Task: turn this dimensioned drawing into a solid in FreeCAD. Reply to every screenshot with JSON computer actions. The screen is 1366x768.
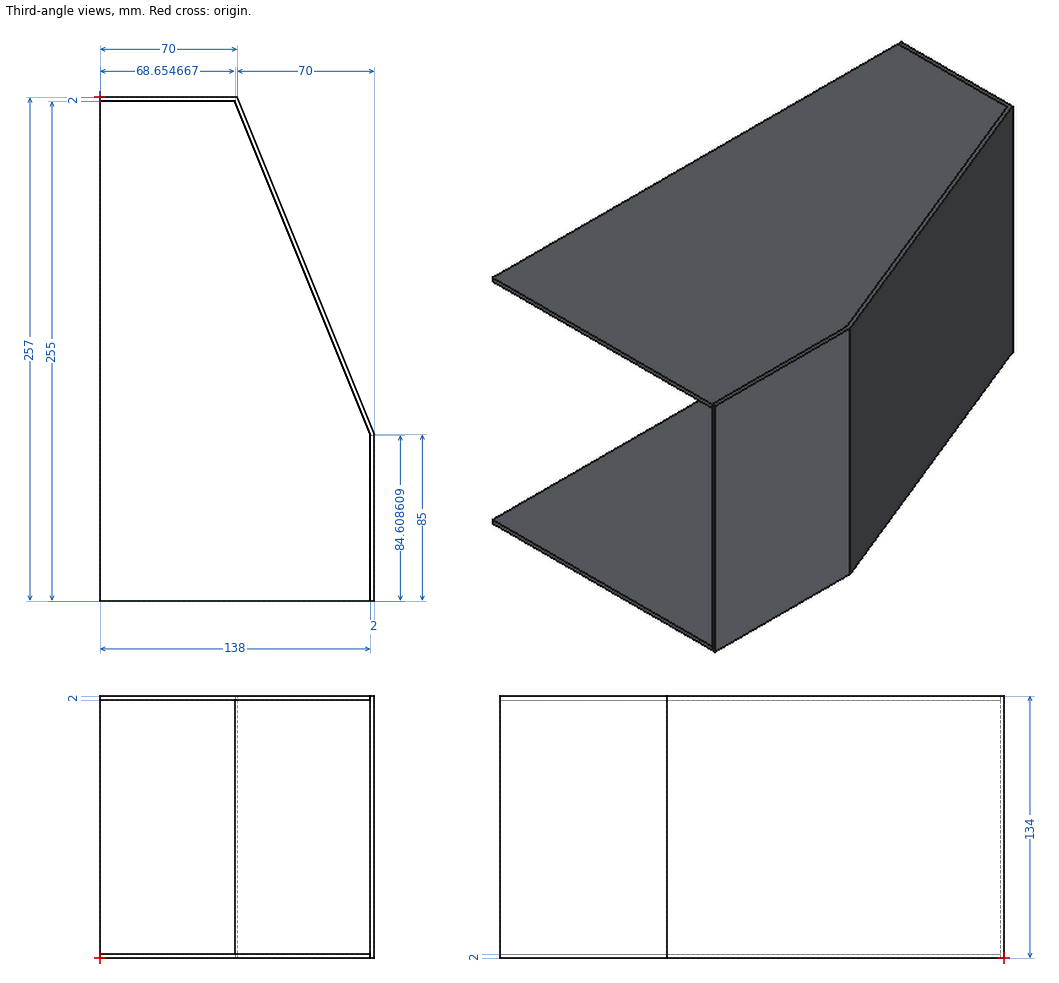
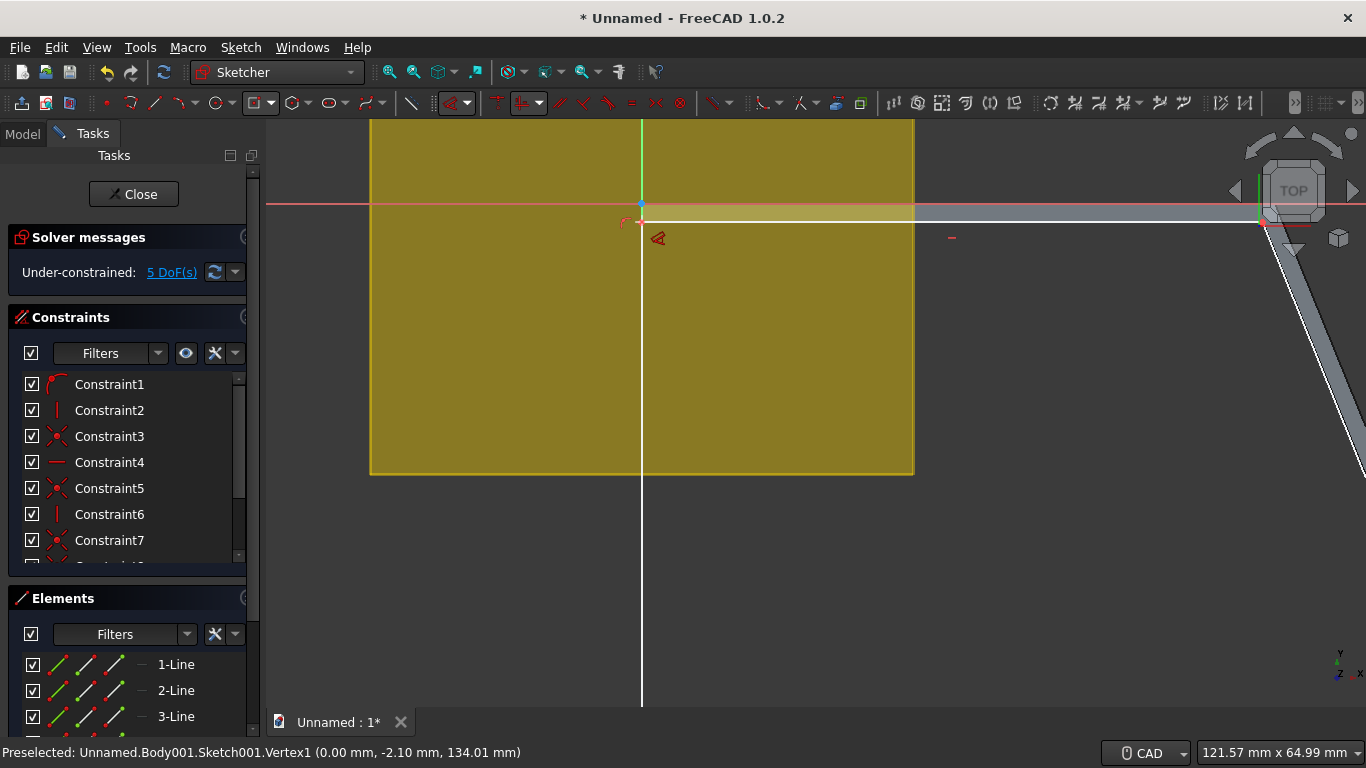
{"action": "scroll", "coordinate": [642, 222], "scroll_direction": "up", "scroll_amount": 4}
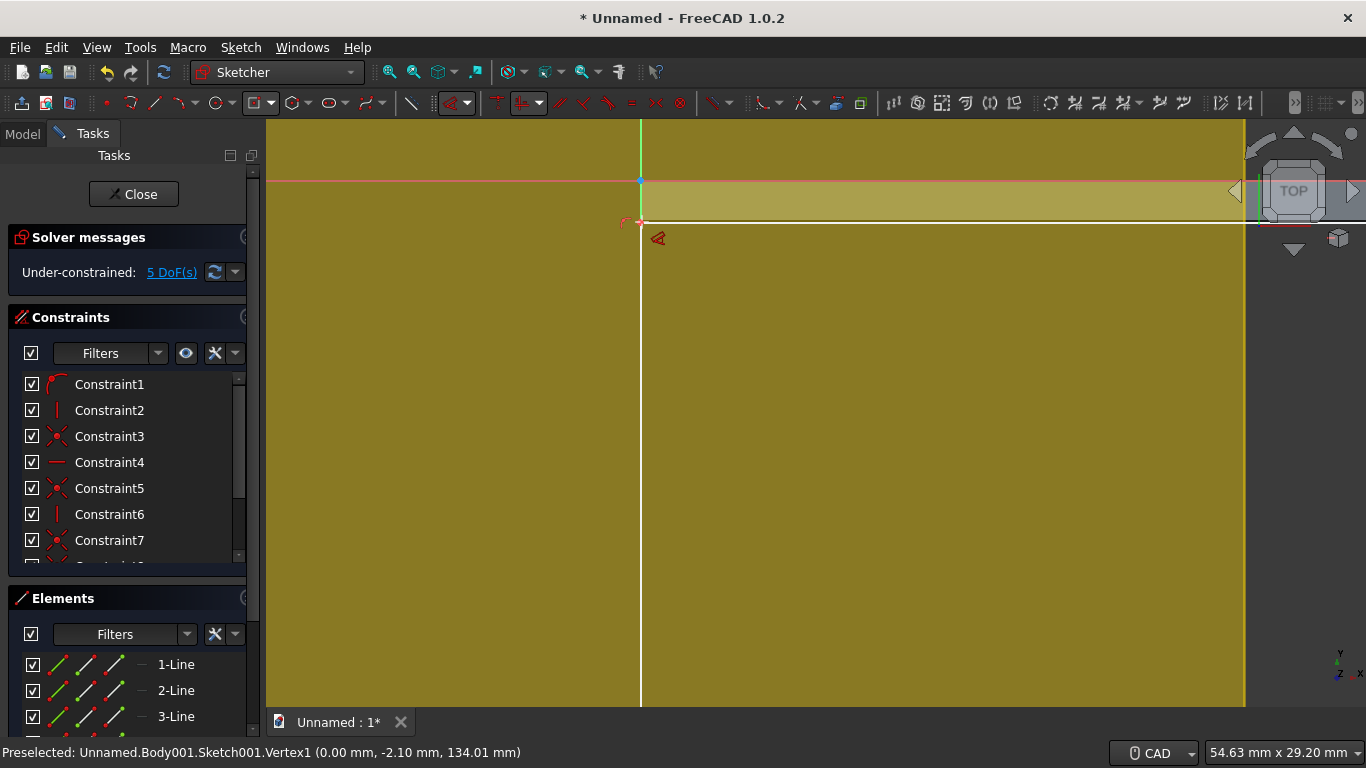
{"action": "left_click", "coordinate": [641, 223]}
{"action": "left_click", "coordinate": [607, 202]}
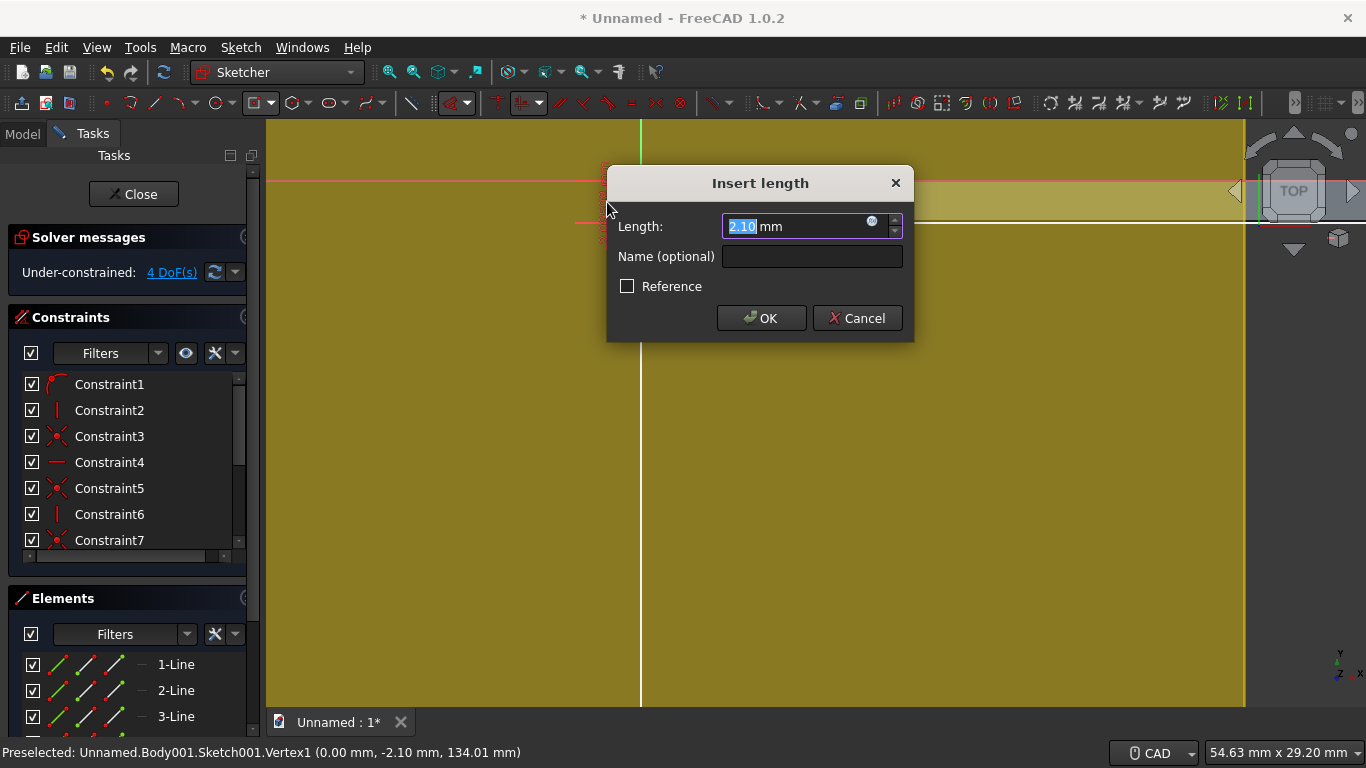
{"action": "type", "text": "2"}
{"action": "key", "text": "Return"}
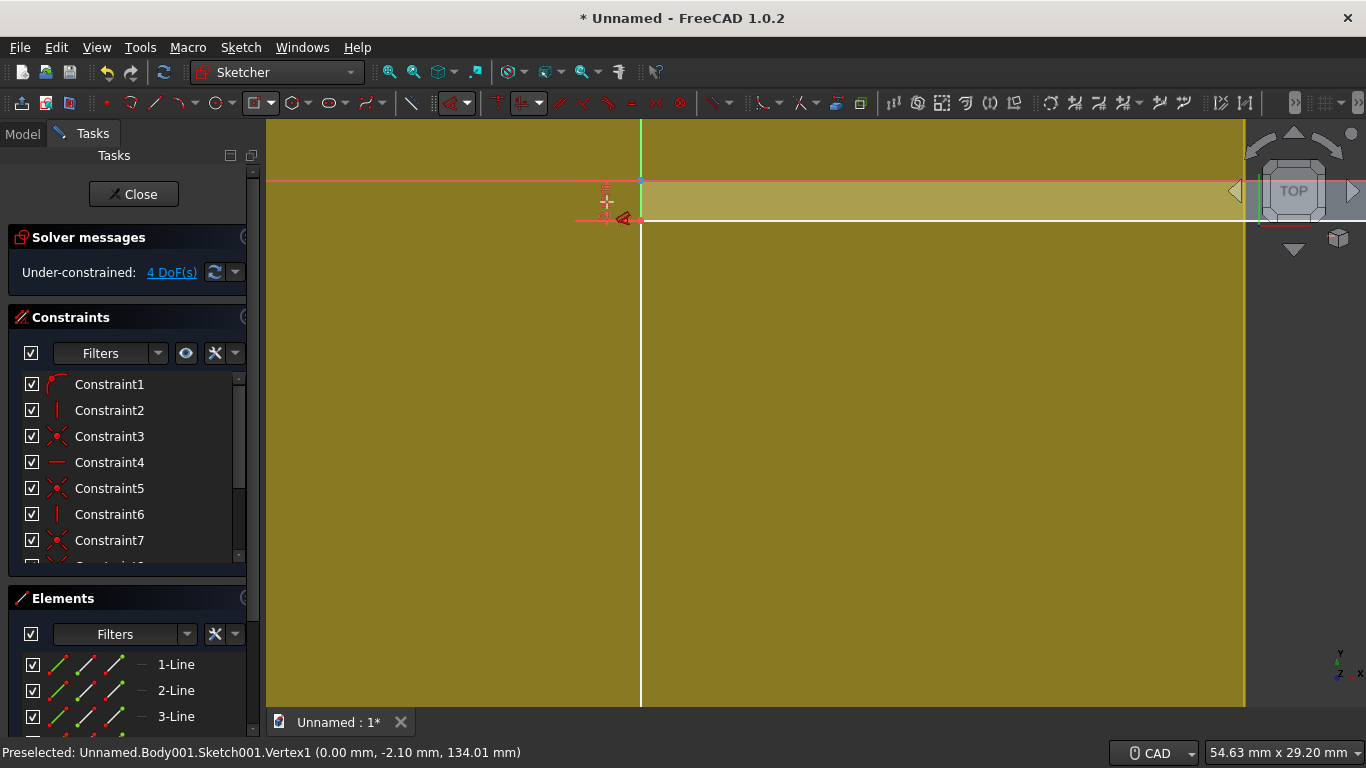
{"action": "scroll", "coordinate": [645, 224], "scroll_direction": "down", "scroll_amount": 13}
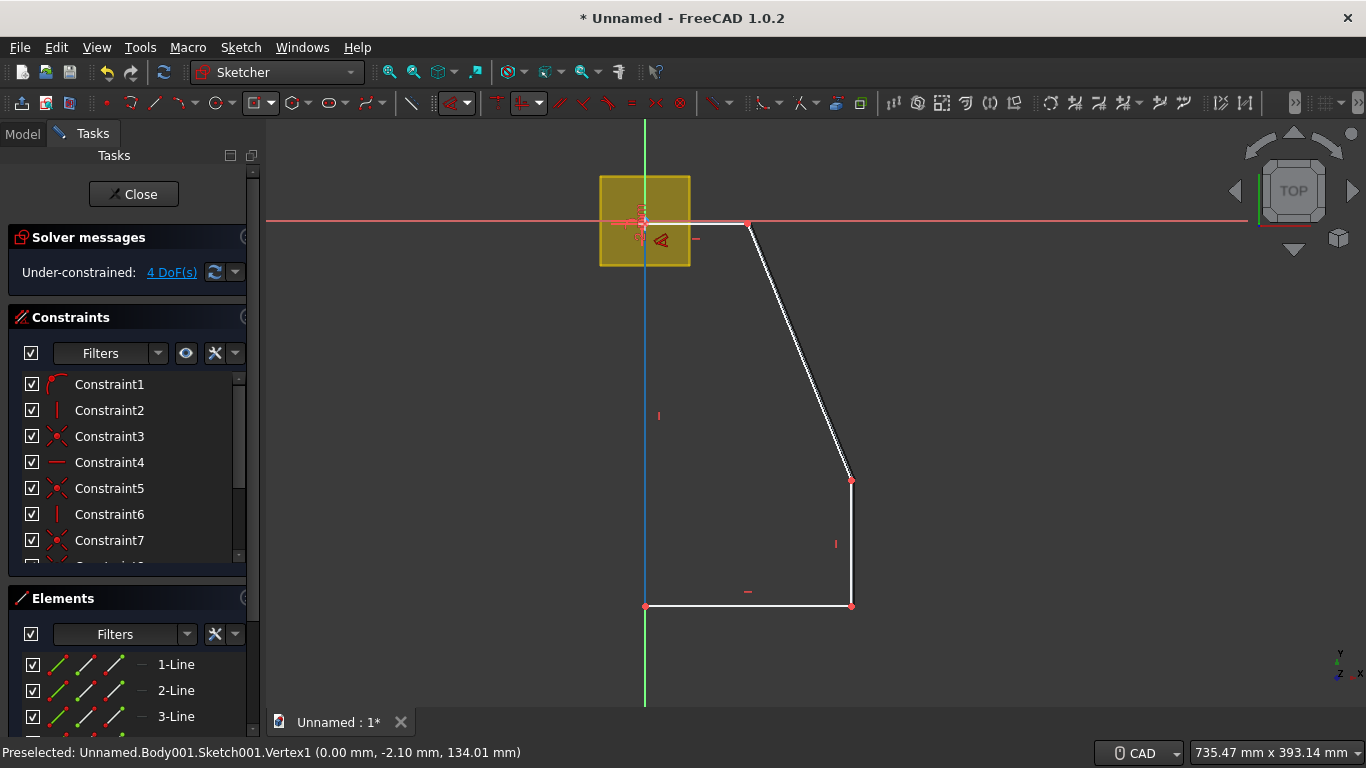
{"action": "left_click", "coordinate": [645, 339]}
{"action": "left_click", "coordinate": [611, 415]}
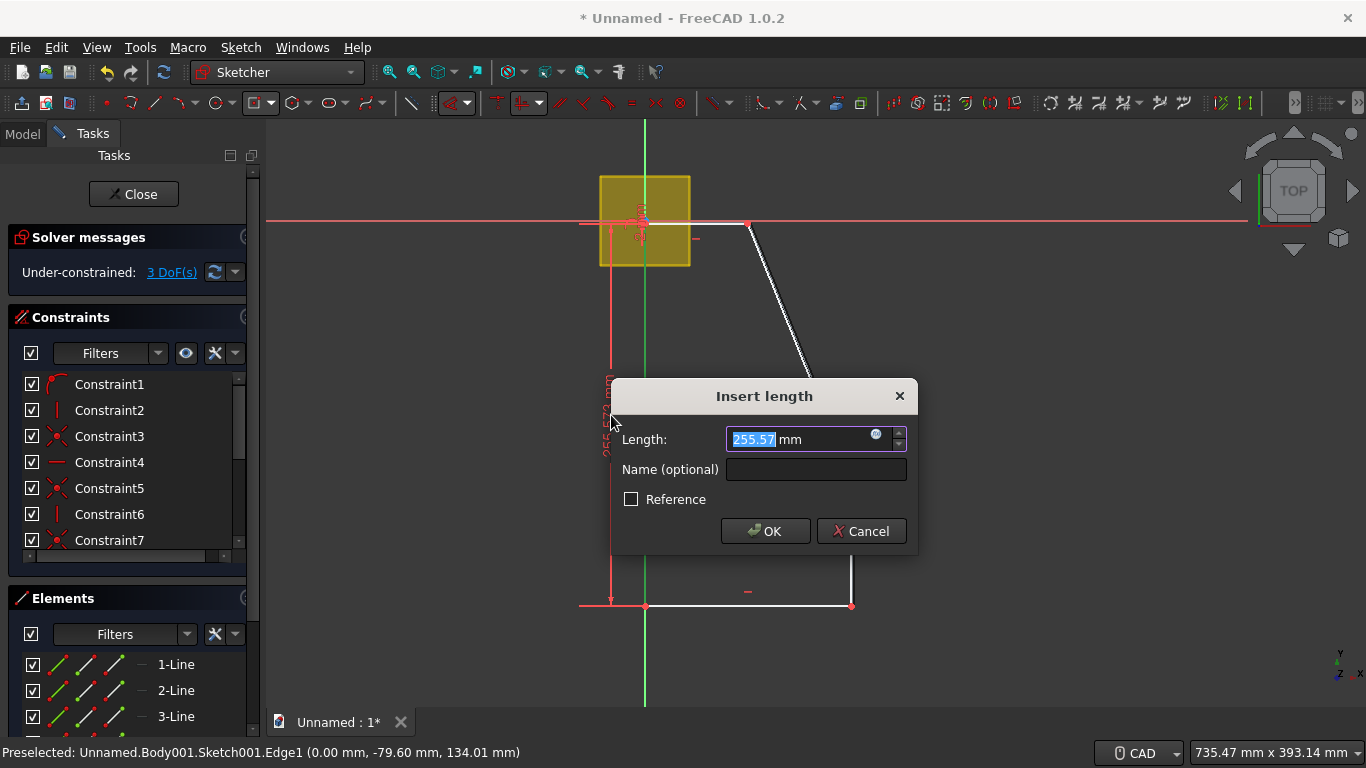
{"action": "type", "text": "255"}
{"action": "key", "text": "Return"}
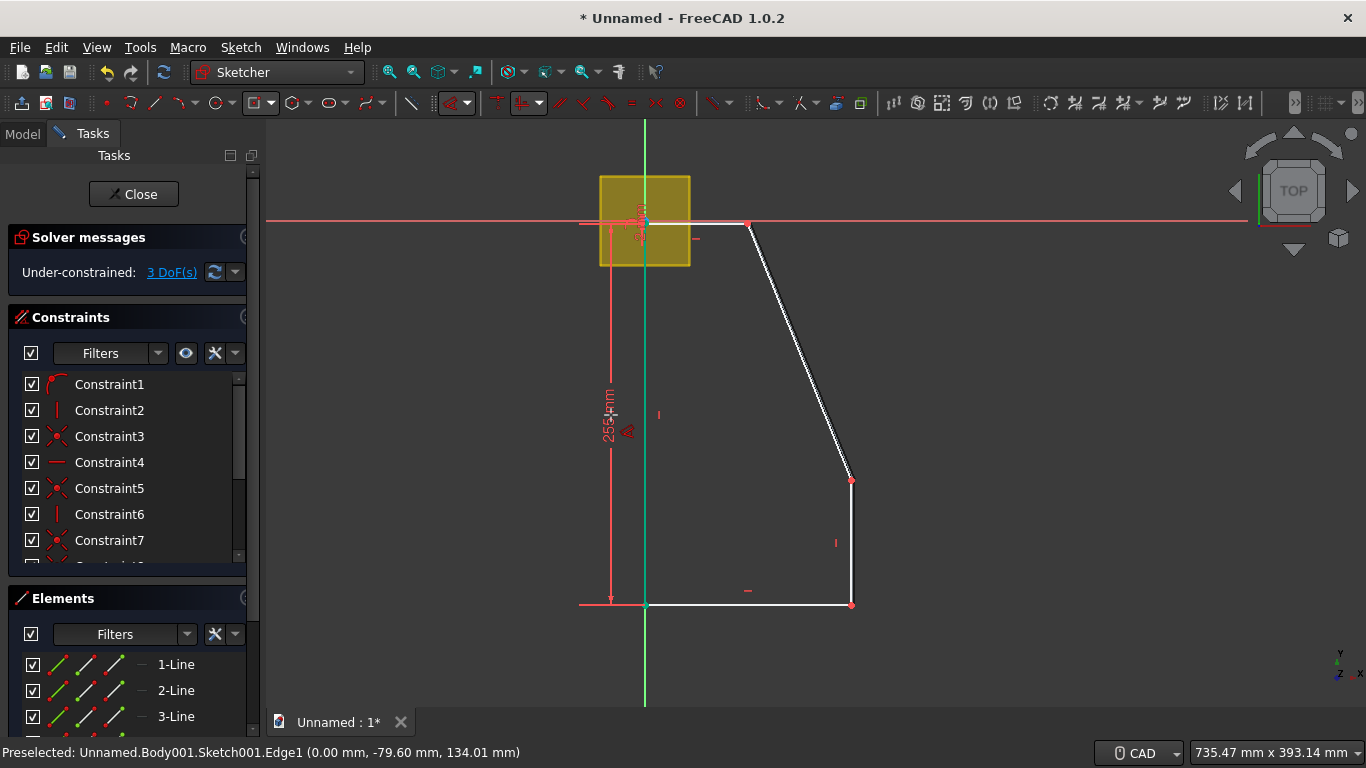
{"action": "left_click", "coordinate": [707, 605]}
{"action": "left_click", "coordinate": [748, 639]}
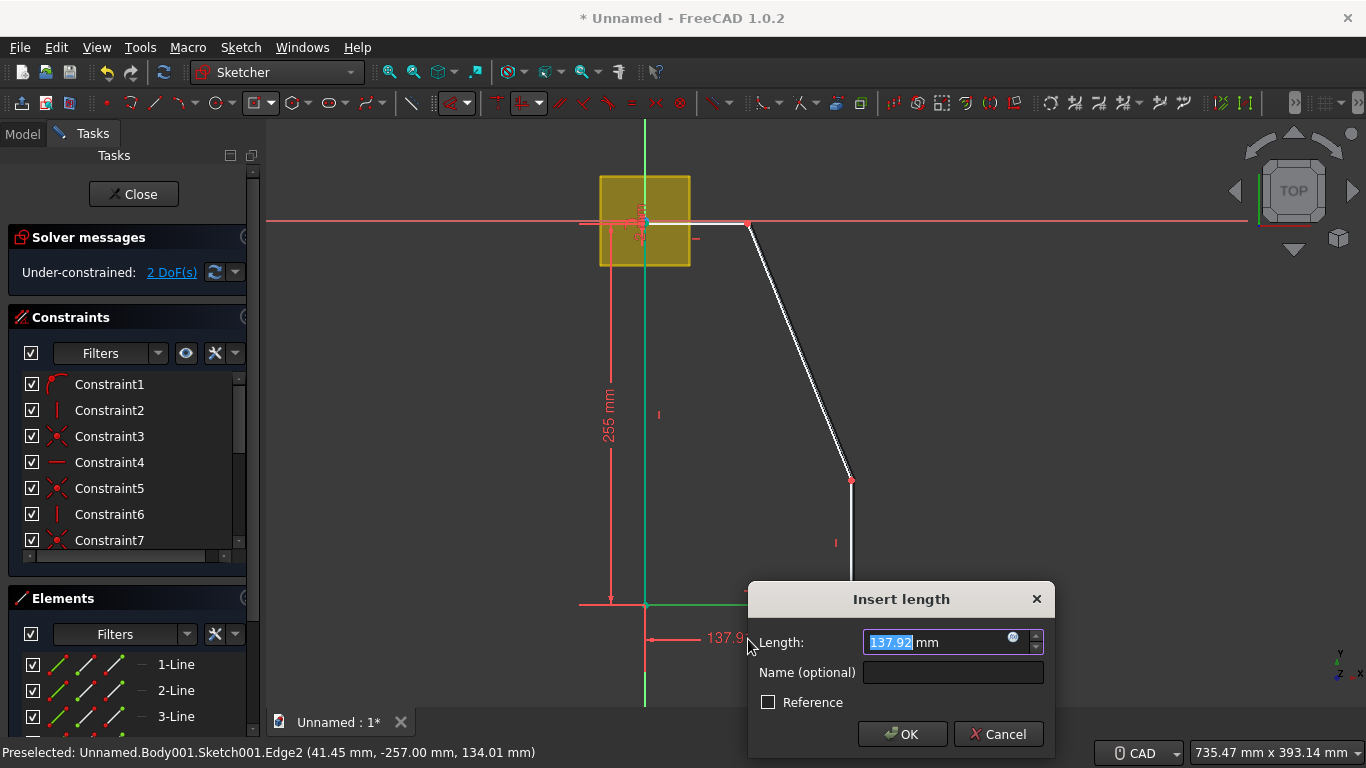
{"action": "type", "text": "138"}
{"action": "key", "text": "Return"}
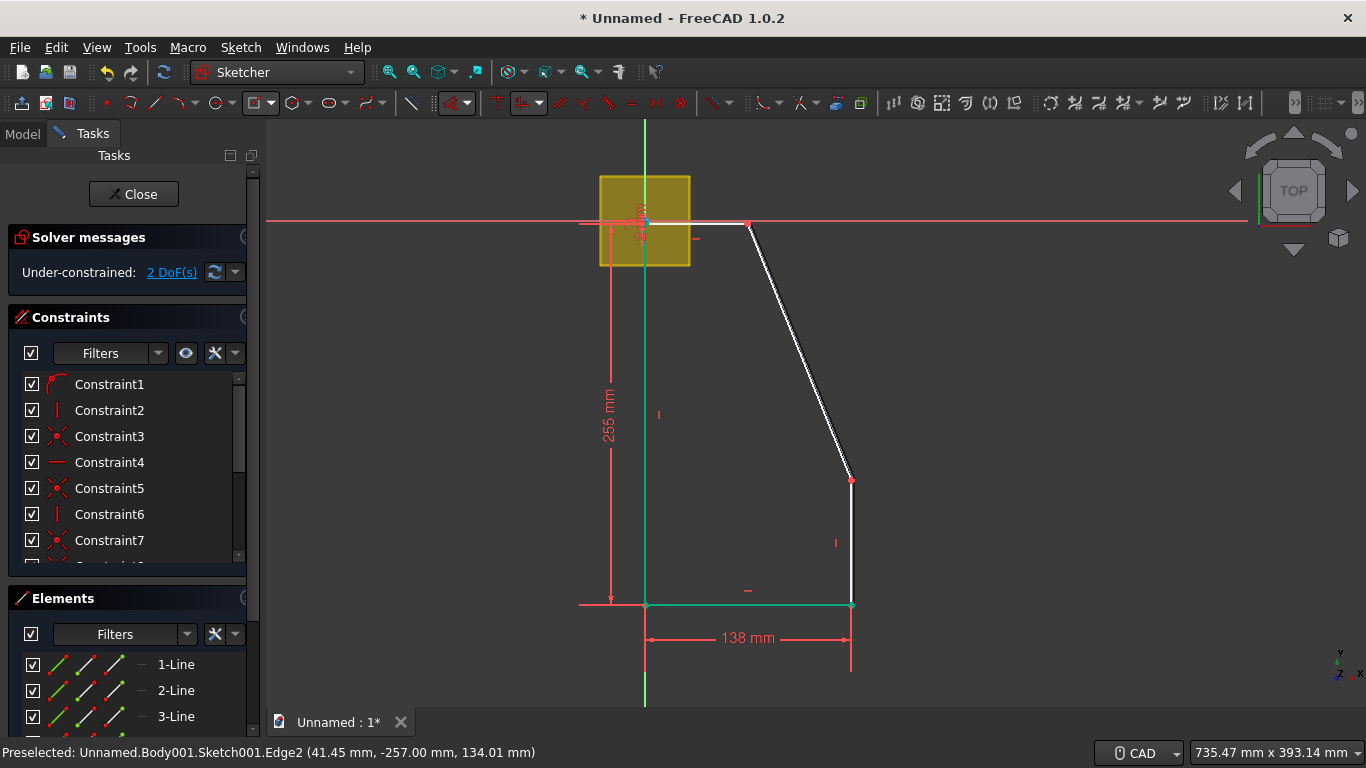
{"action": "left_click", "coordinate": [851, 568]}
{"action": "left_click", "coordinate": [885, 543]}